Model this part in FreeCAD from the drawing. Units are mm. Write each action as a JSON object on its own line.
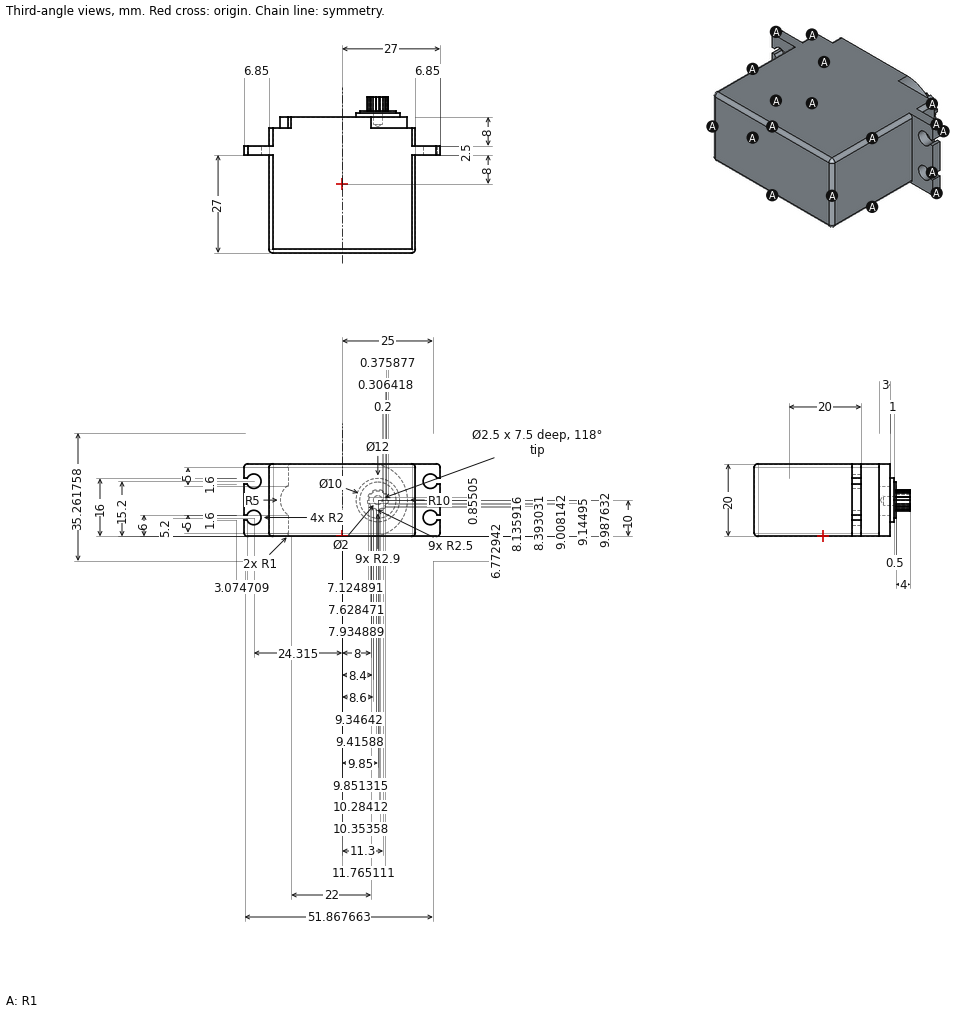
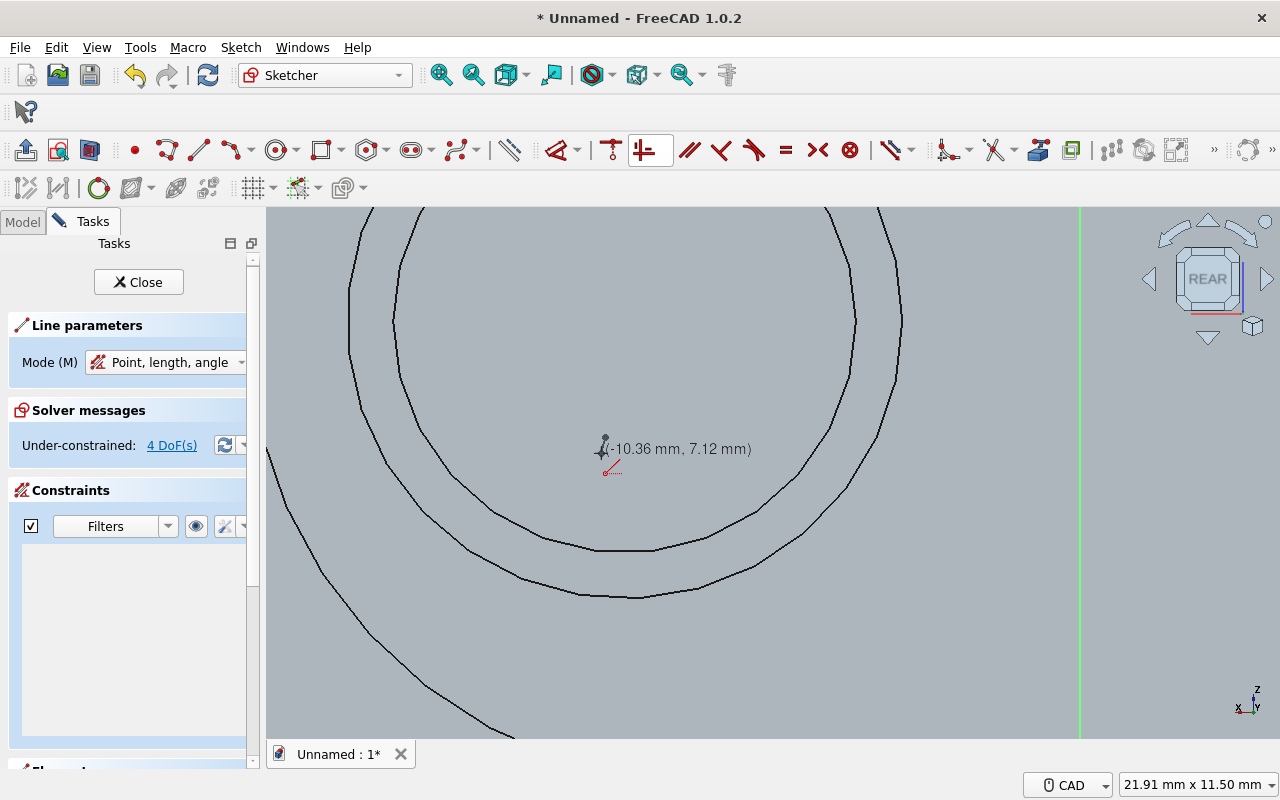
{"action": "left_click", "coordinate": [648, 453]}
{"action": "left_click", "coordinate": [645, 435]}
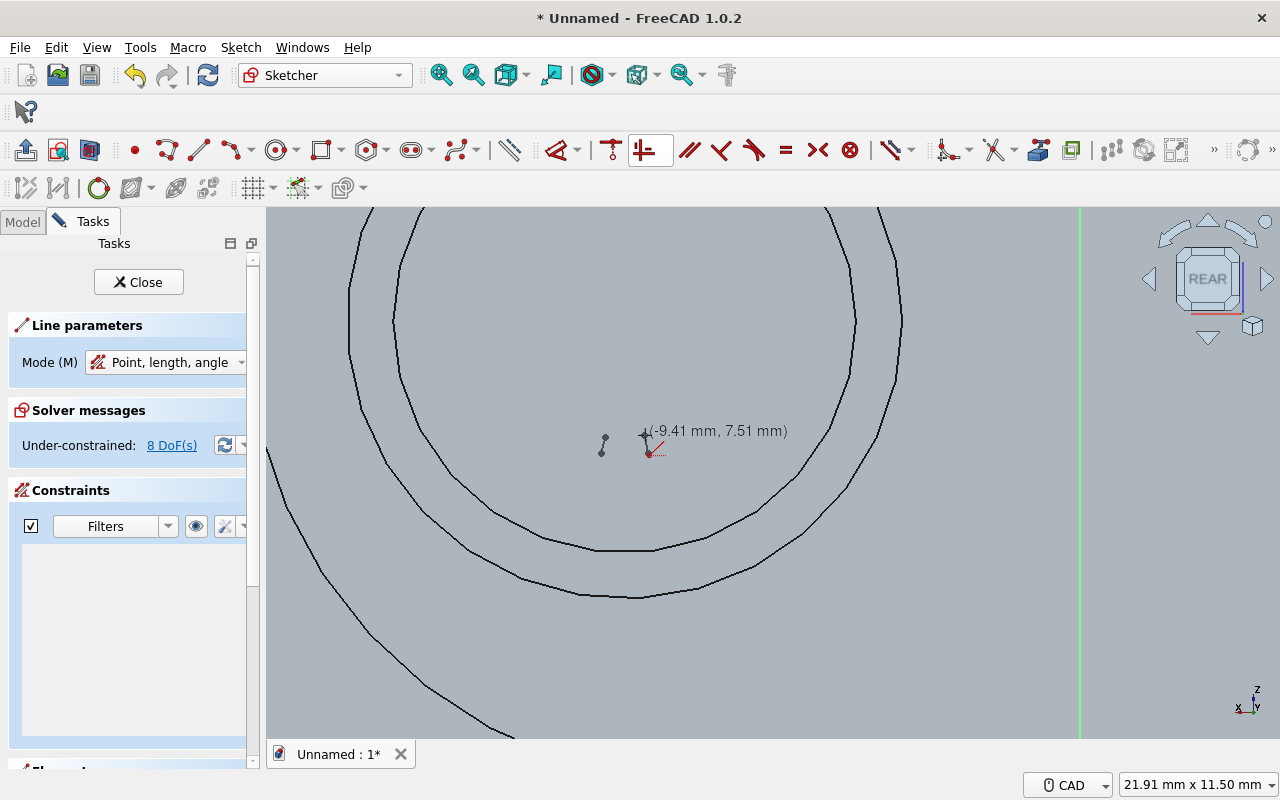
{"action": "left_click", "coordinate": [682, 421]}
{"action": "left_click", "coordinate": [692, 437]}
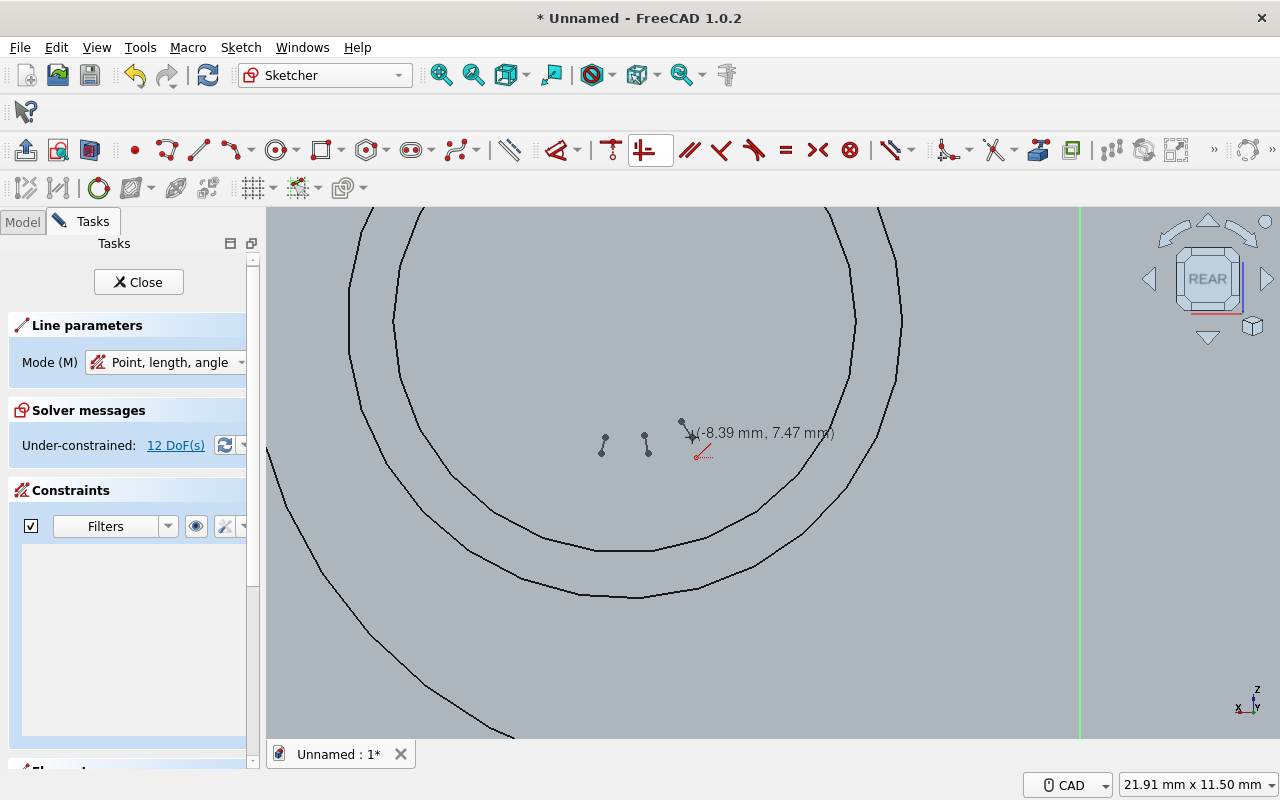
{"action": "left_click", "coordinate": [727, 407]}
{"action": "left_click", "coordinate": [713, 395]}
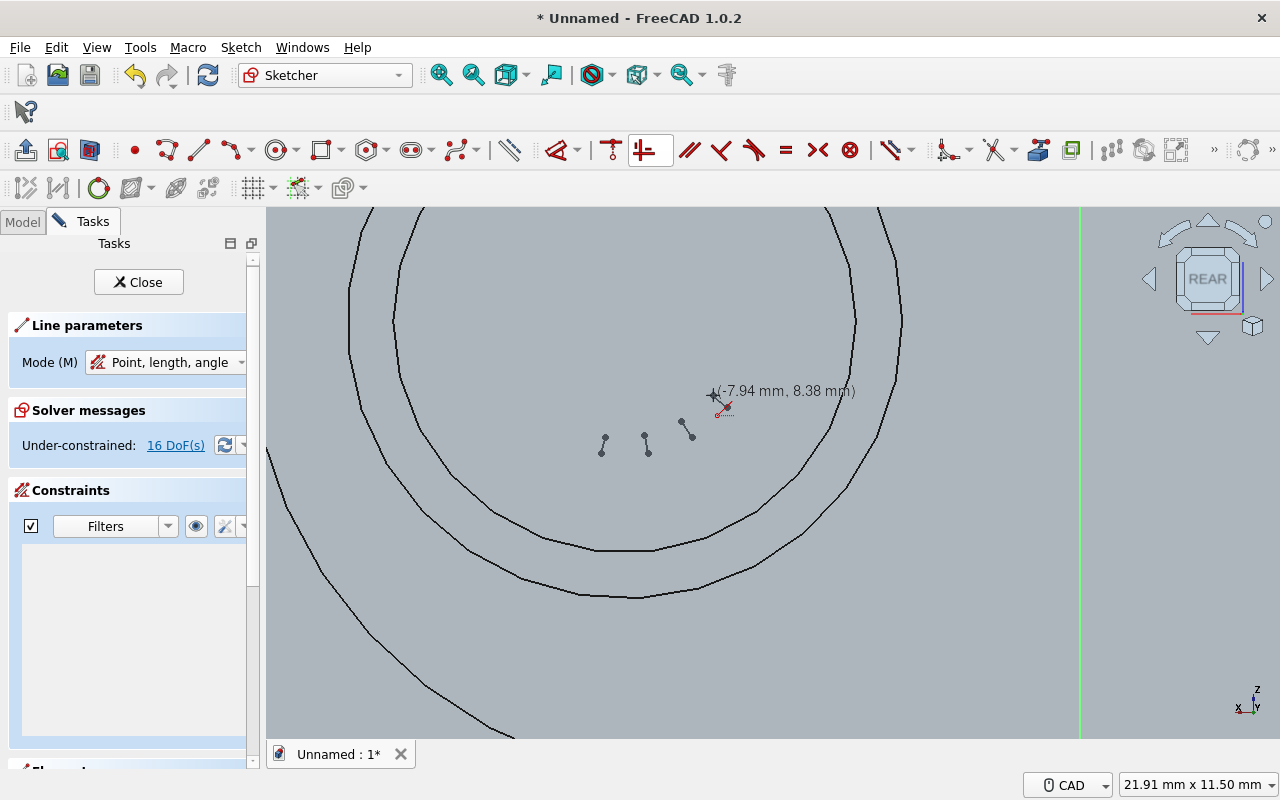
{"action": "left_click", "coordinate": [733, 361]}
{"action": "left_click", "coordinate": [751, 367]}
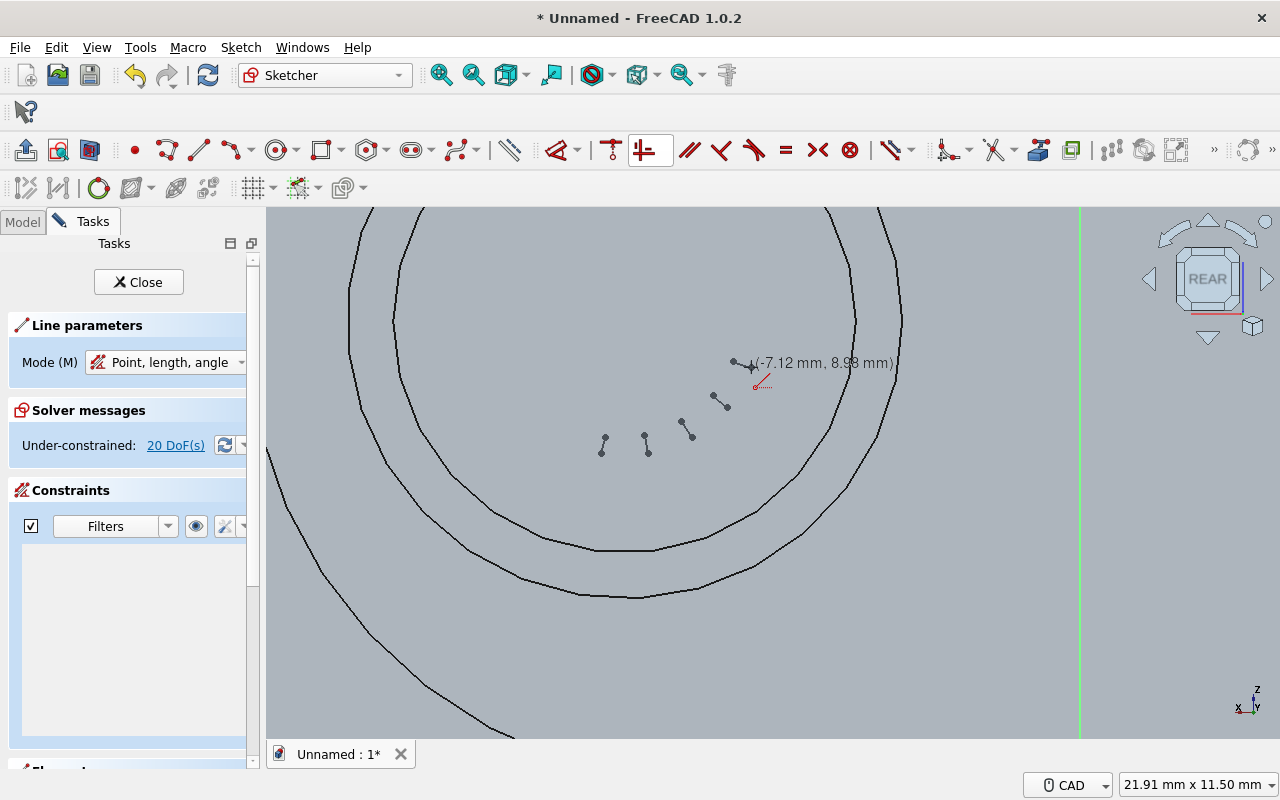
{"action": "left_click", "coordinate": [759, 321]}
{"action": "left_click", "coordinate": [740, 321]}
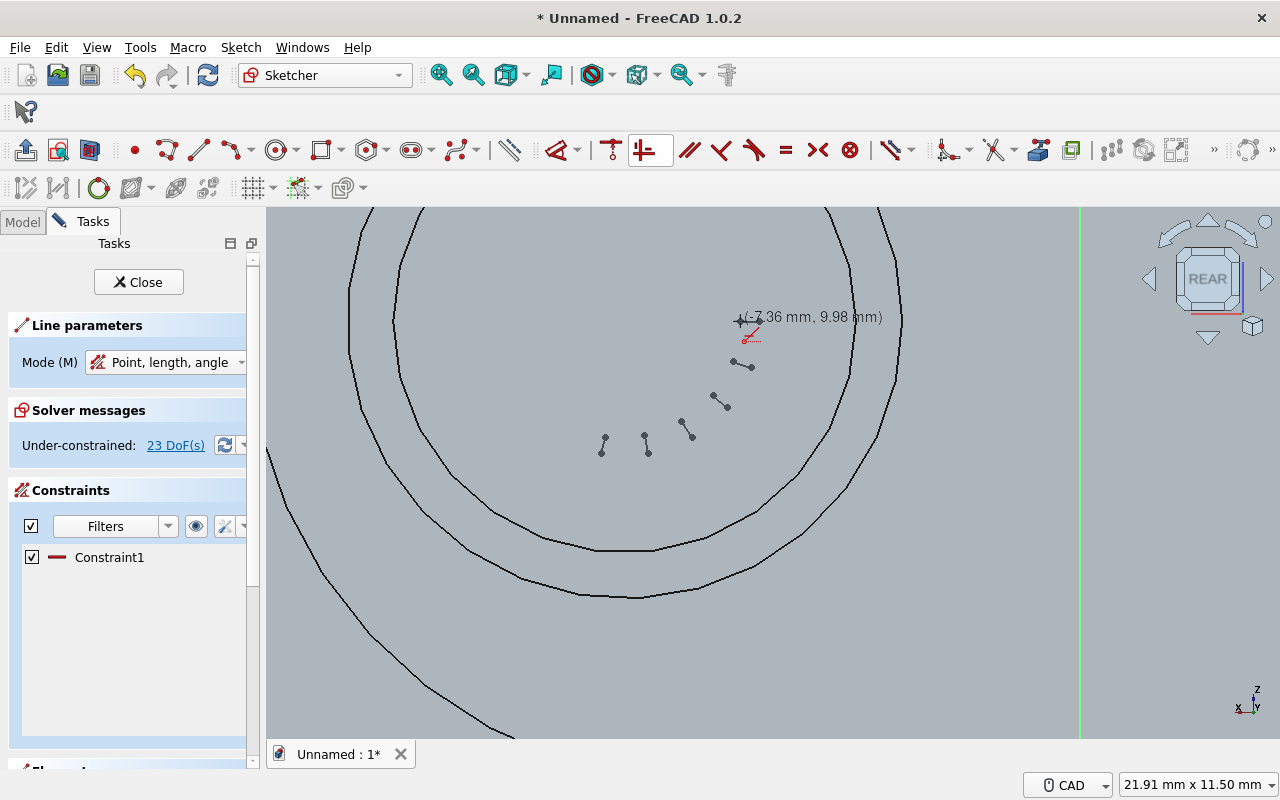
{"action": "left_click", "coordinate": [733, 281]}
{"action": "left_click", "coordinate": [751, 275]}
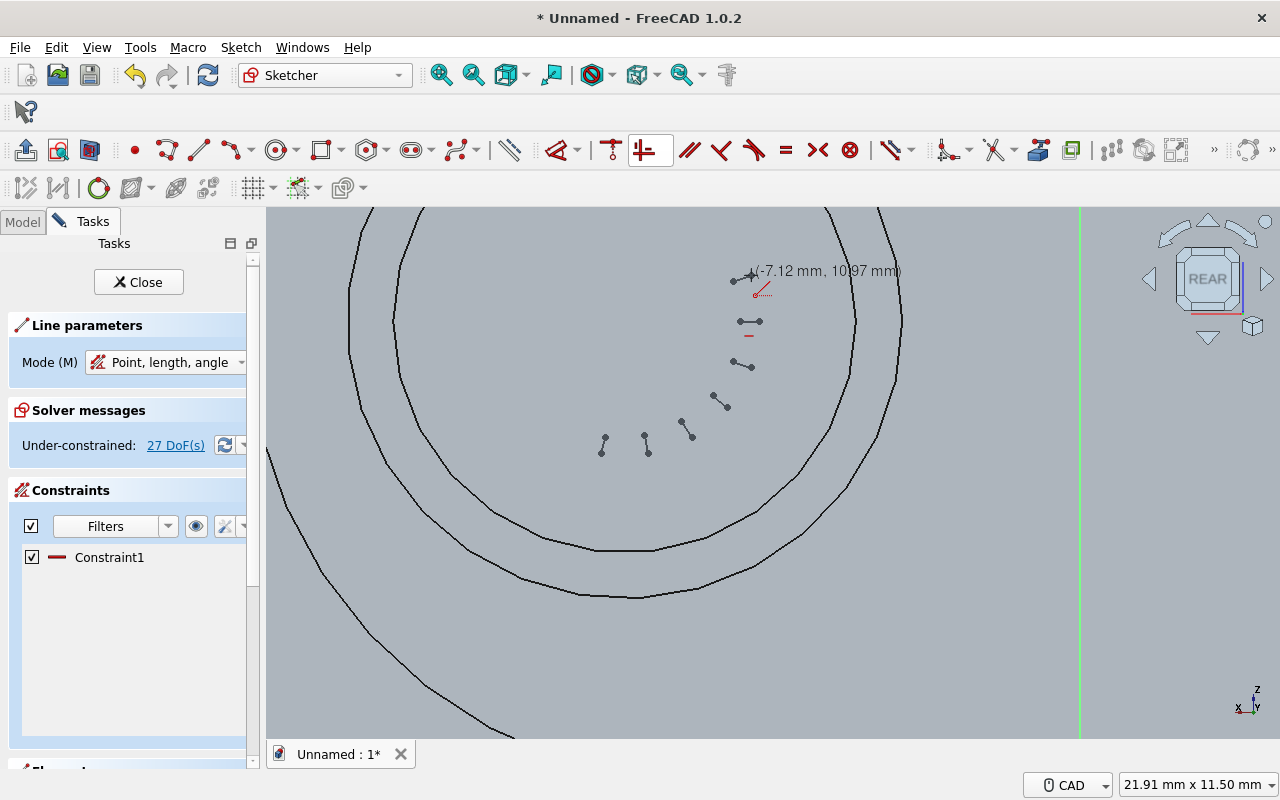
{"action": "scroll", "coordinate": [606, 457], "scroll_direction": "down", "scroll_amount": 3}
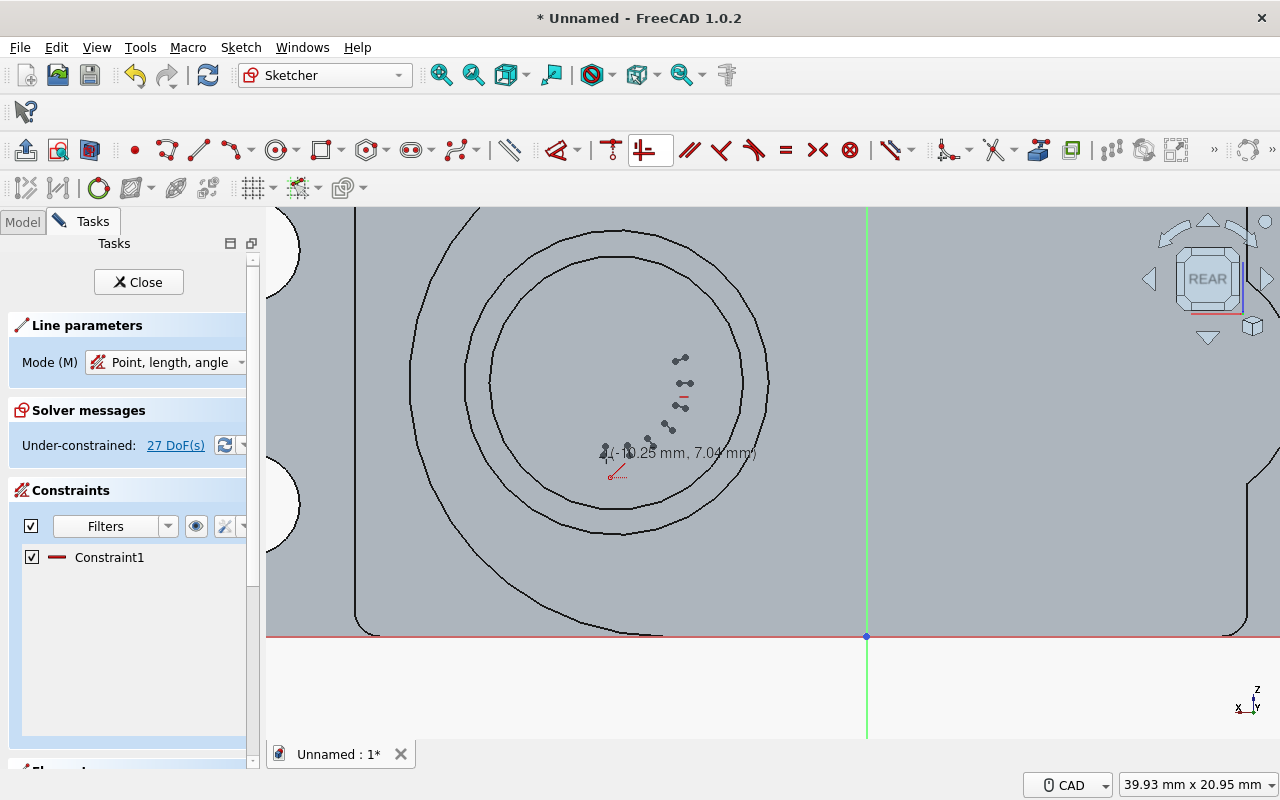
{"action": "left_click", "coordinate": [673, 335]}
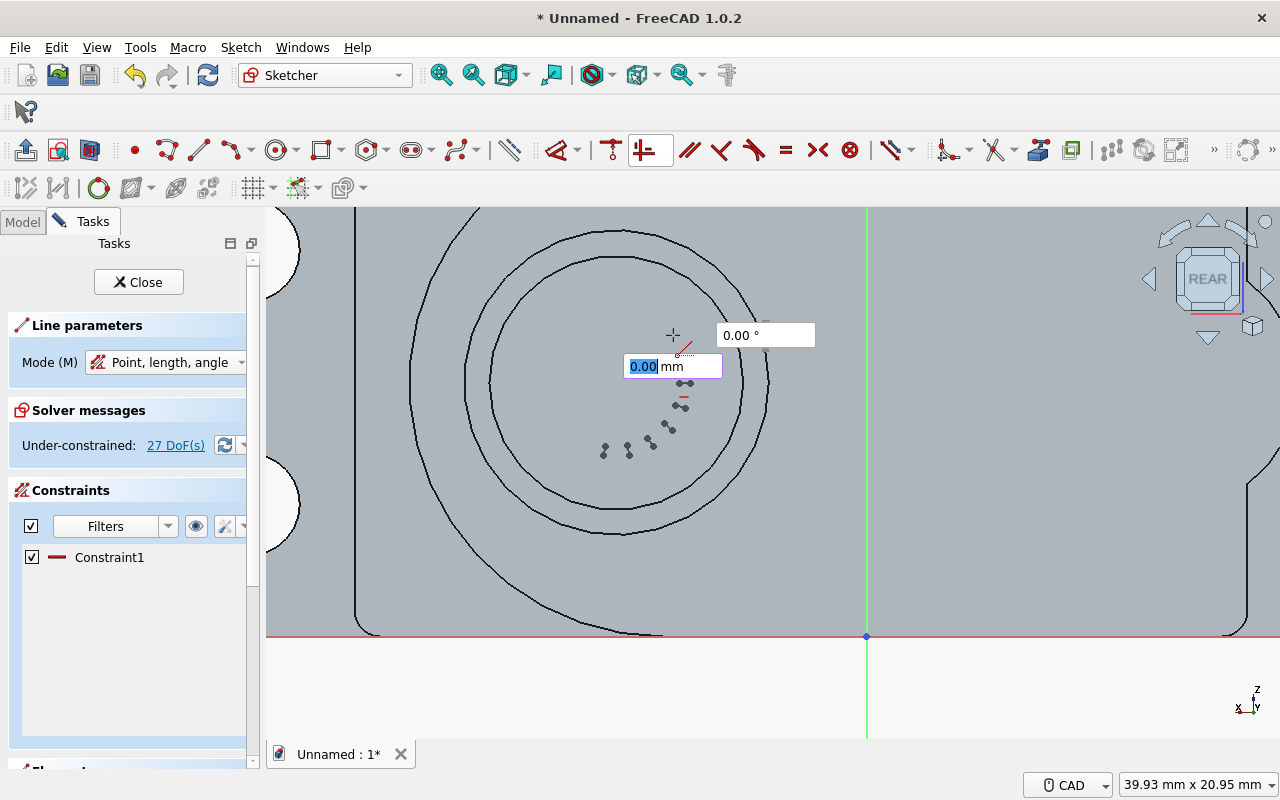
{"action": "scroll", "coordinate": [665, 342], "scroll_direction": "up", "scroll_amount": 3}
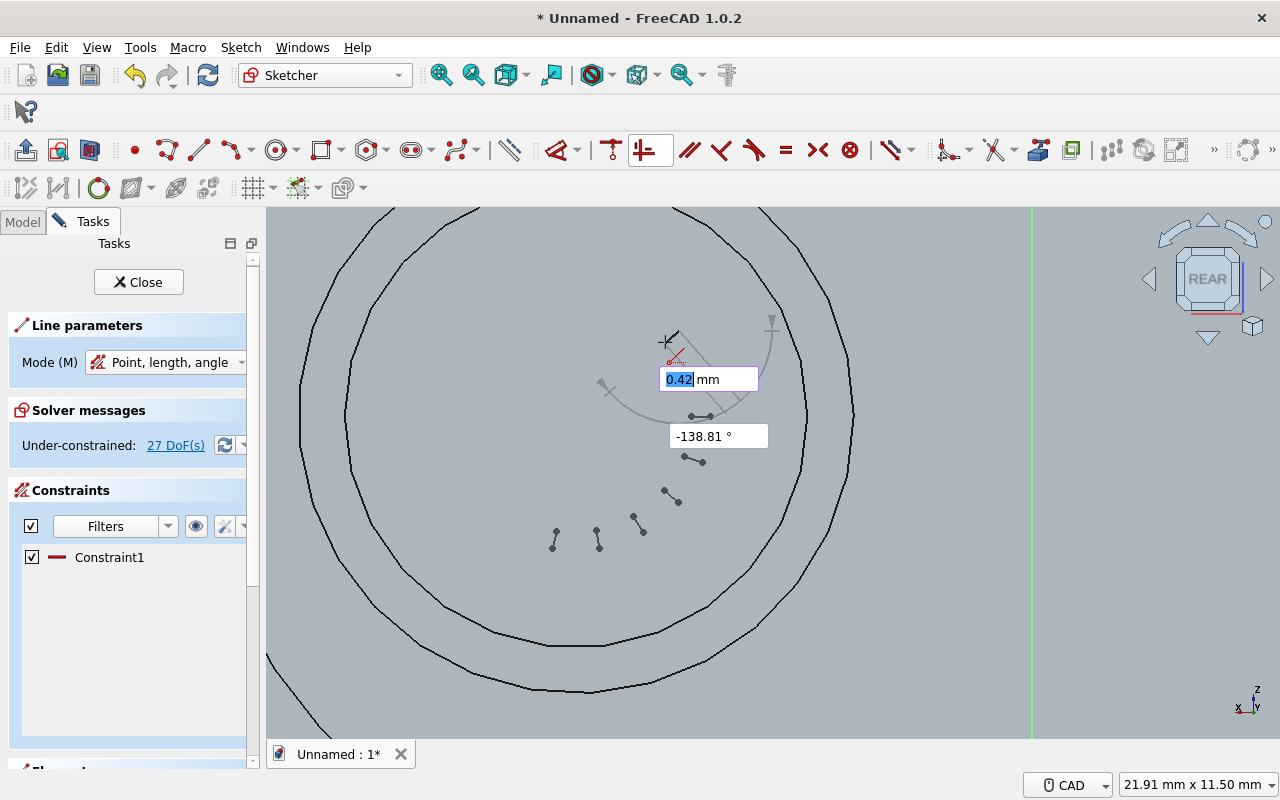
{"action": "left_click", "coordinate": [665, 341]}